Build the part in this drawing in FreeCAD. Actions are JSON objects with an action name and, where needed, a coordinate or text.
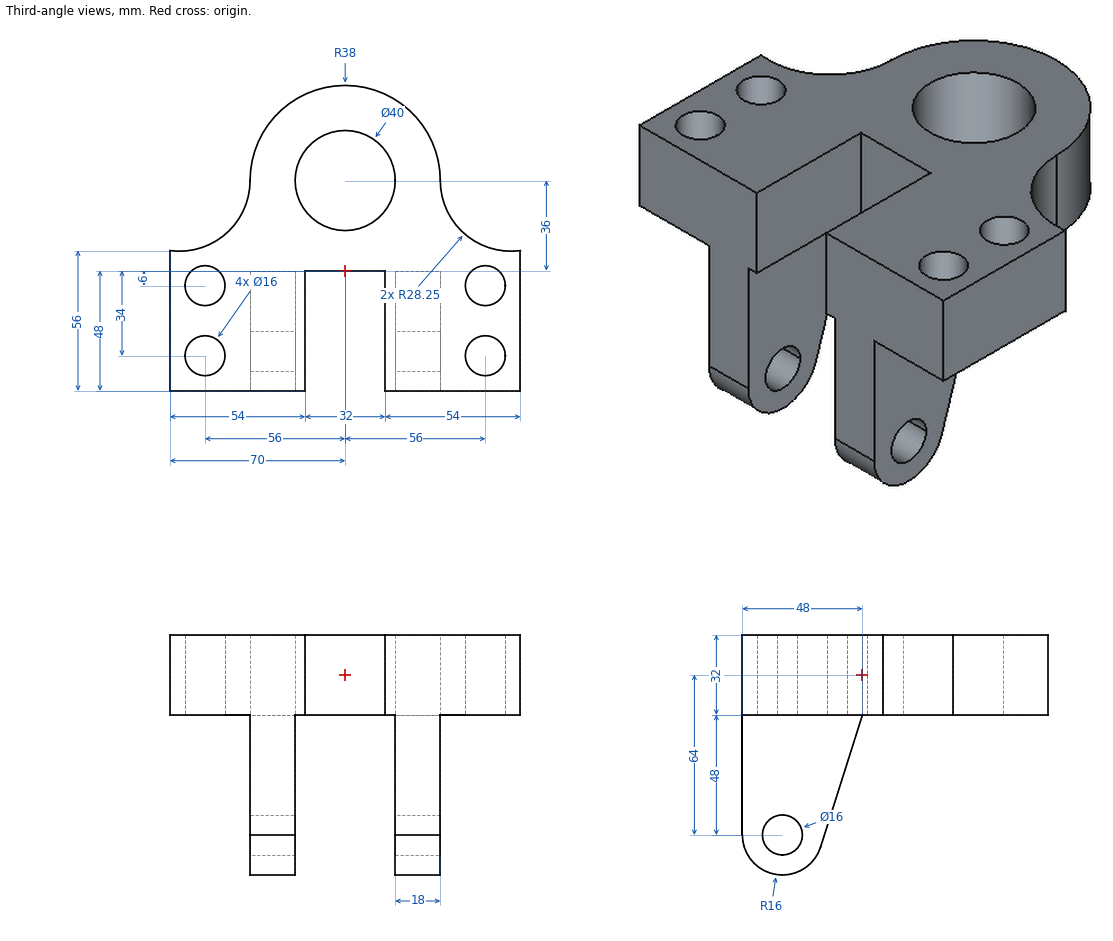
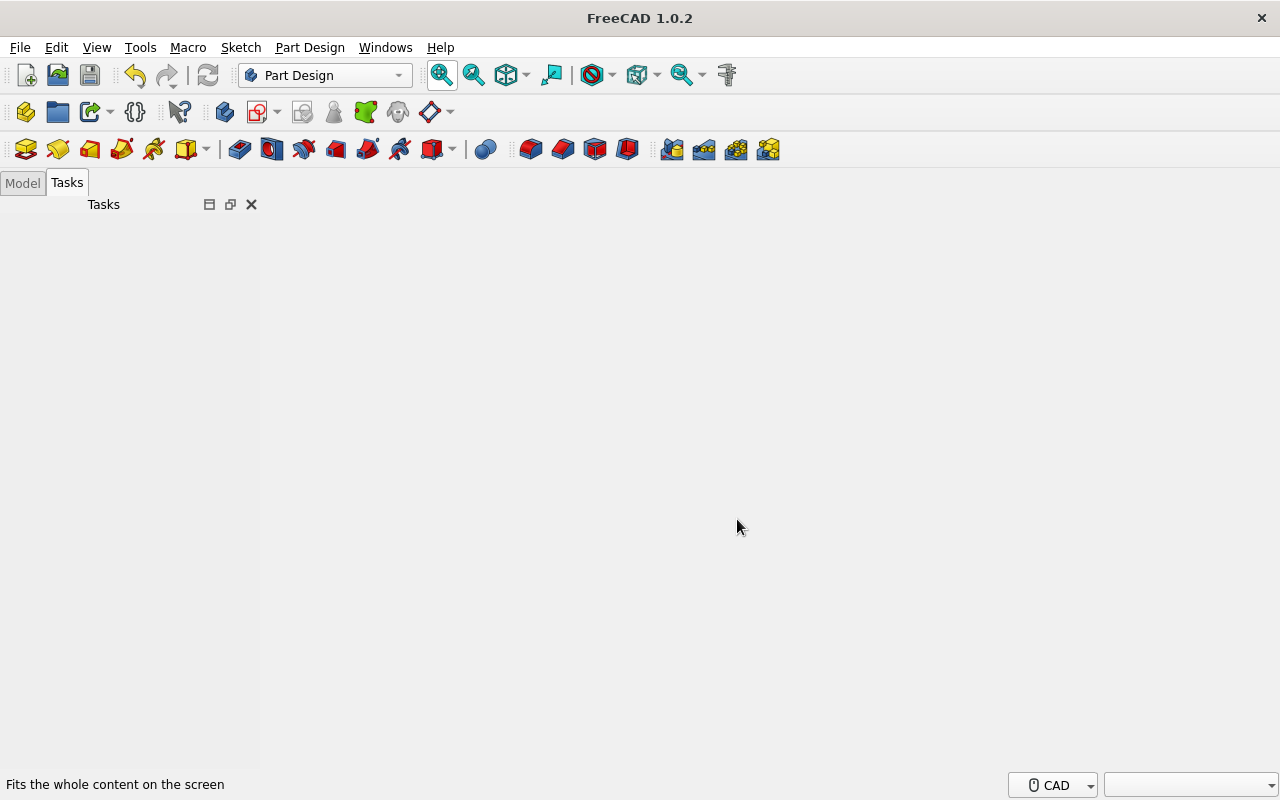
{"action": "left_click", "coordinate": [26, 76]}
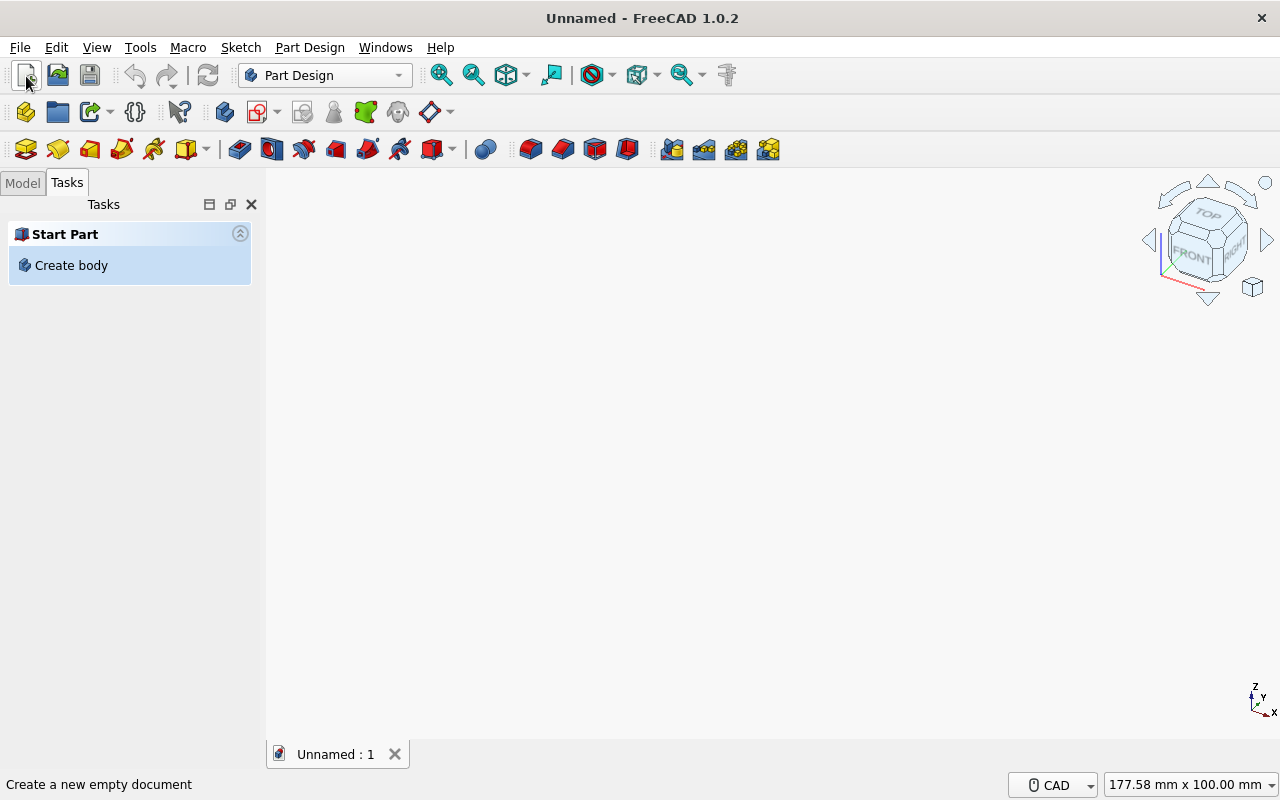
{"action": "left_click", "coordinate": [258, 112]}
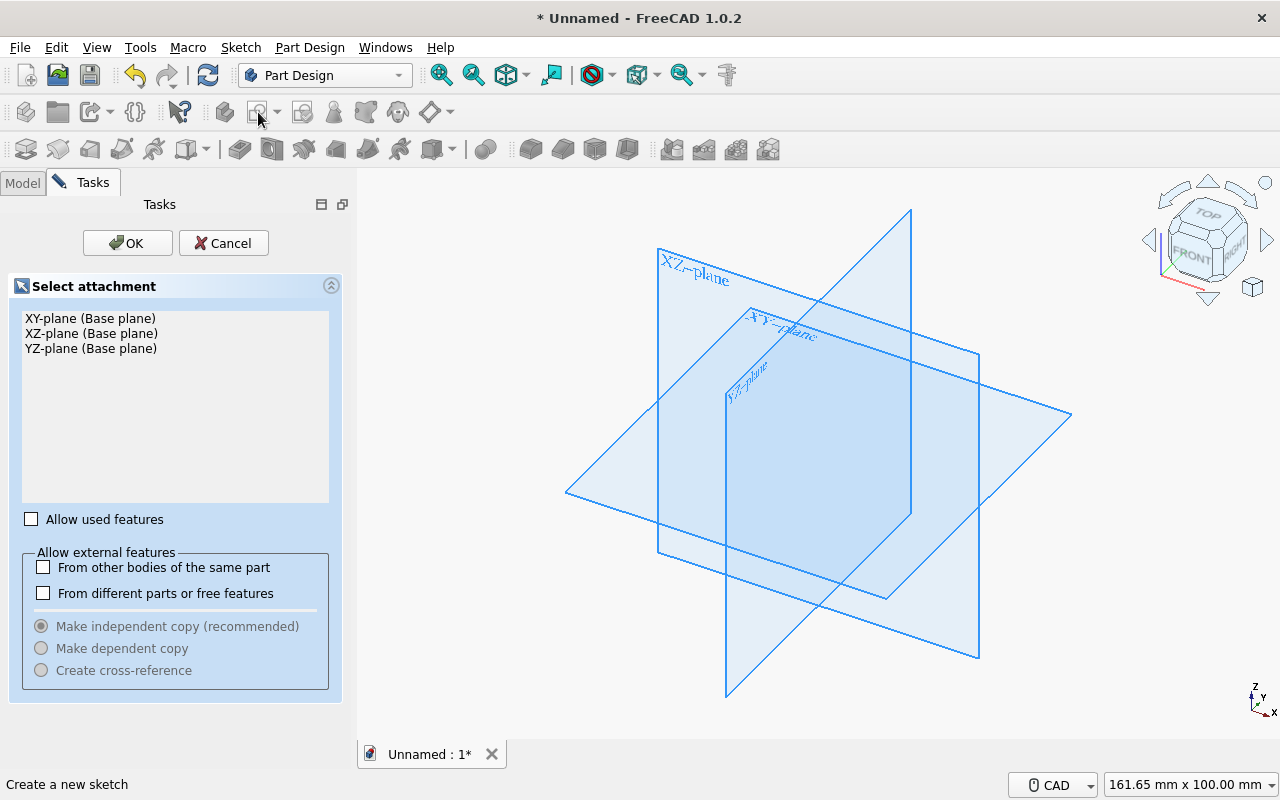
{"action": "left_click", "coordinate": [82, 318]}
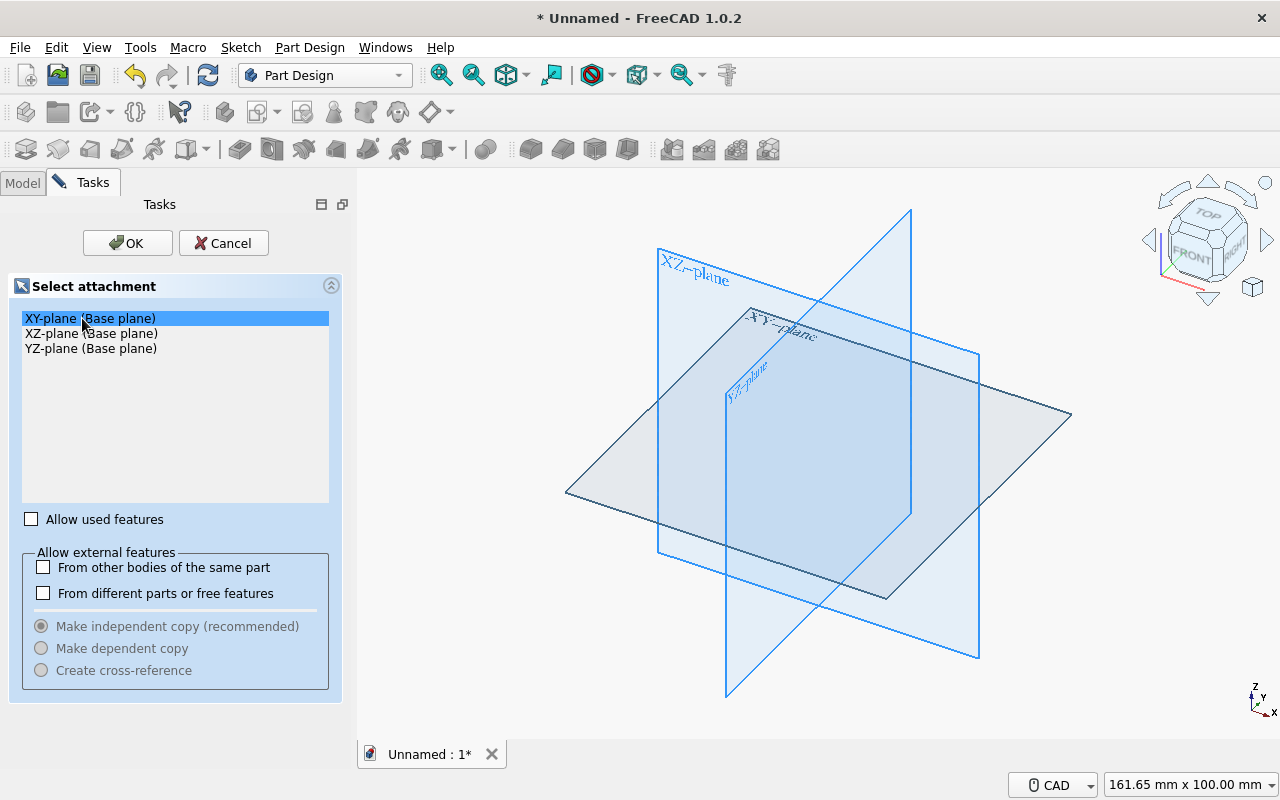
{"action": "left_click", "coordinate": [128, 243]}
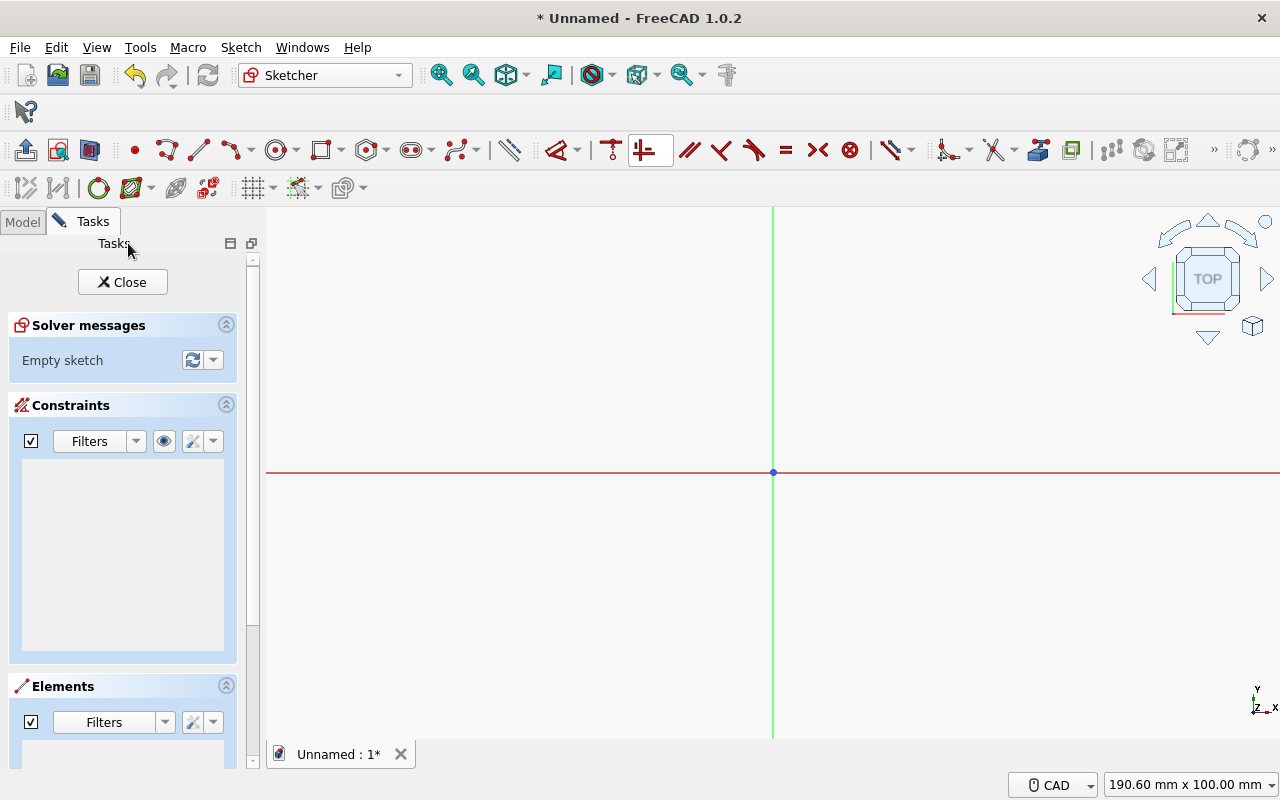
{"action": "scroll", "coordinate": [621, 557], "scroll_direction": "down", "scroll_amount": 3}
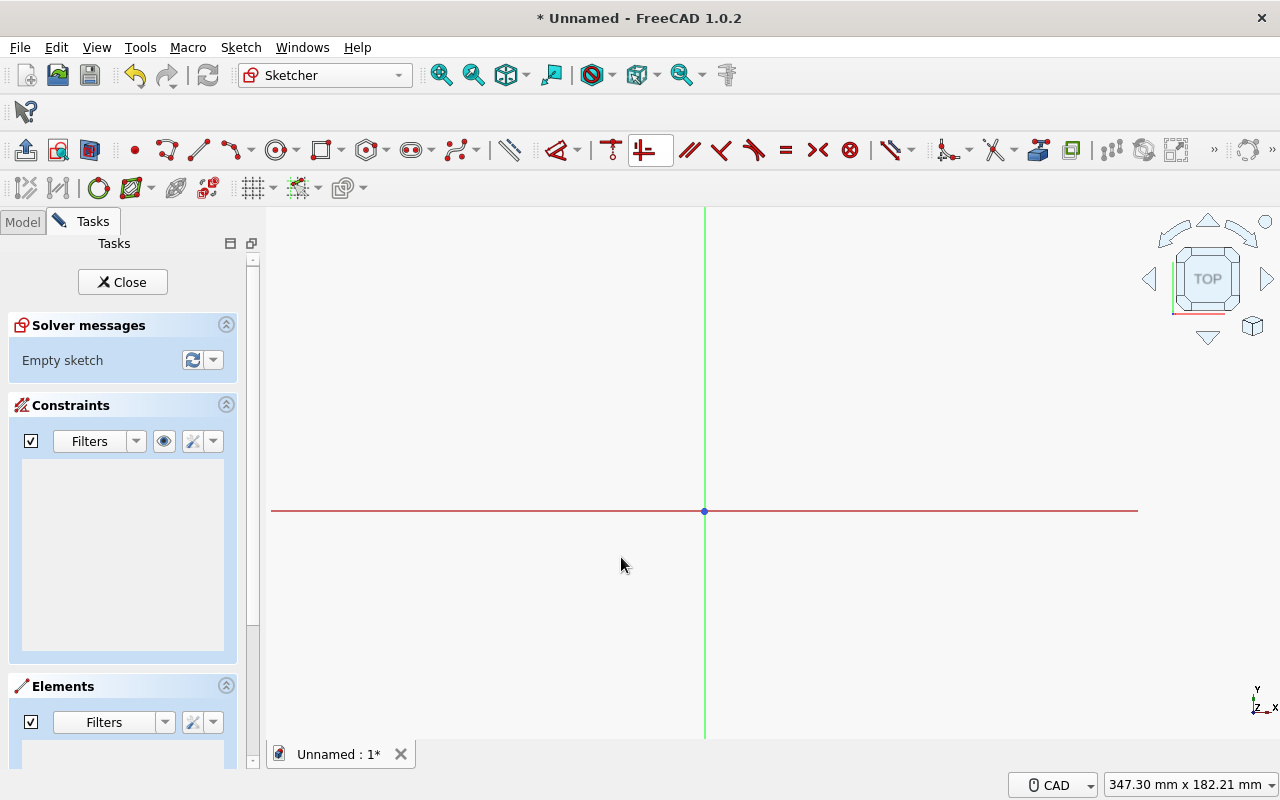
{"action": "left_click", "coordinate": [168, 150]}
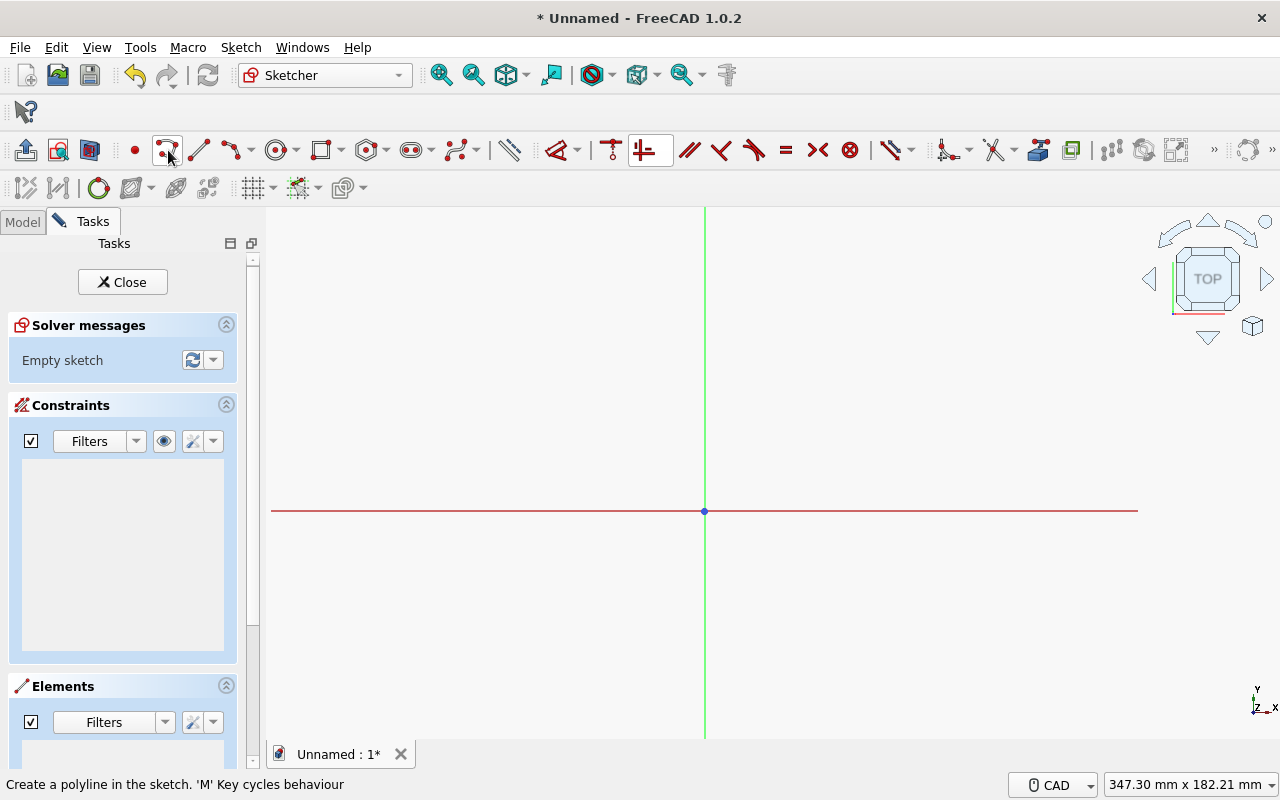
{"action": "left_click", "coordinate": [500, 488]}
{"action": "left_click", "coordinate": [500, 651]}
{"action": "left_click", "coordinate": [658, 651]}
{"action": "left_click", "coordinate": [658, 511]}
{"action": "left_click", "coordinate": [751, 502]}
{"action": "left_click", "coordinate": [751, 651]}
{"action": "left_click", "coordinate": [909, 651]}
{"action": "left_click", "coordinate": [909, 488]}
{"action": "right_click", "coordinate": [909, 488]}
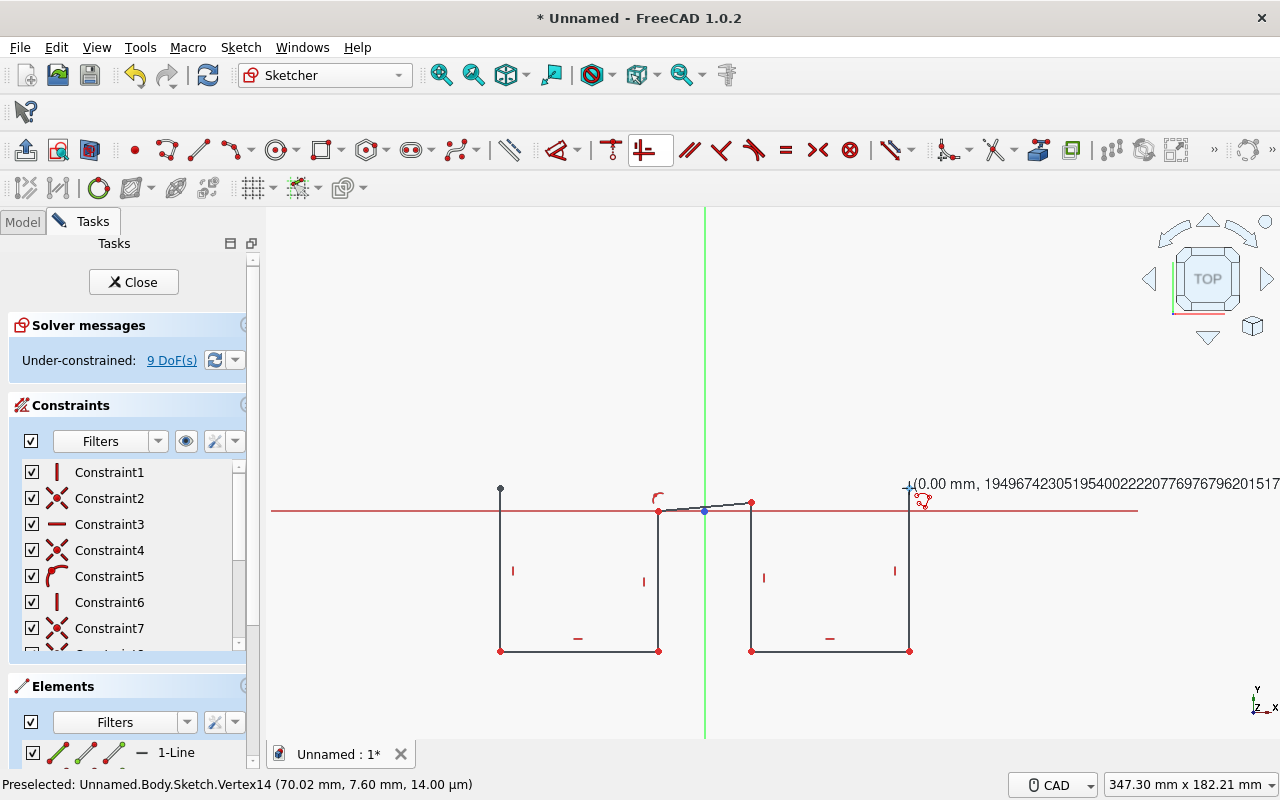
{"action": "left_click", "coordinate": [232, 150]}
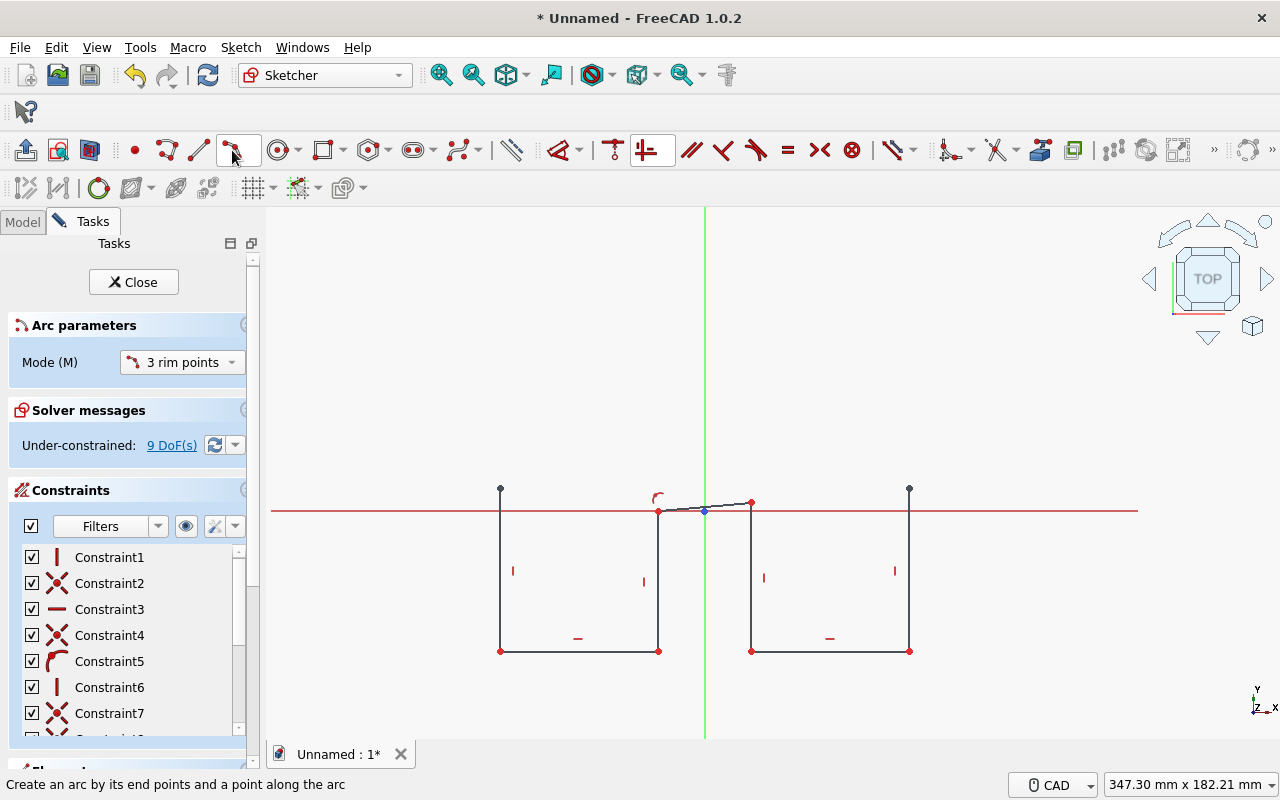
{"action": "left_click", "coordinate": [909, 489]}
{"action": "left_click", "coordinate": [816, 406]}
{"action": "left_click", "coordinate": [844, 468]}